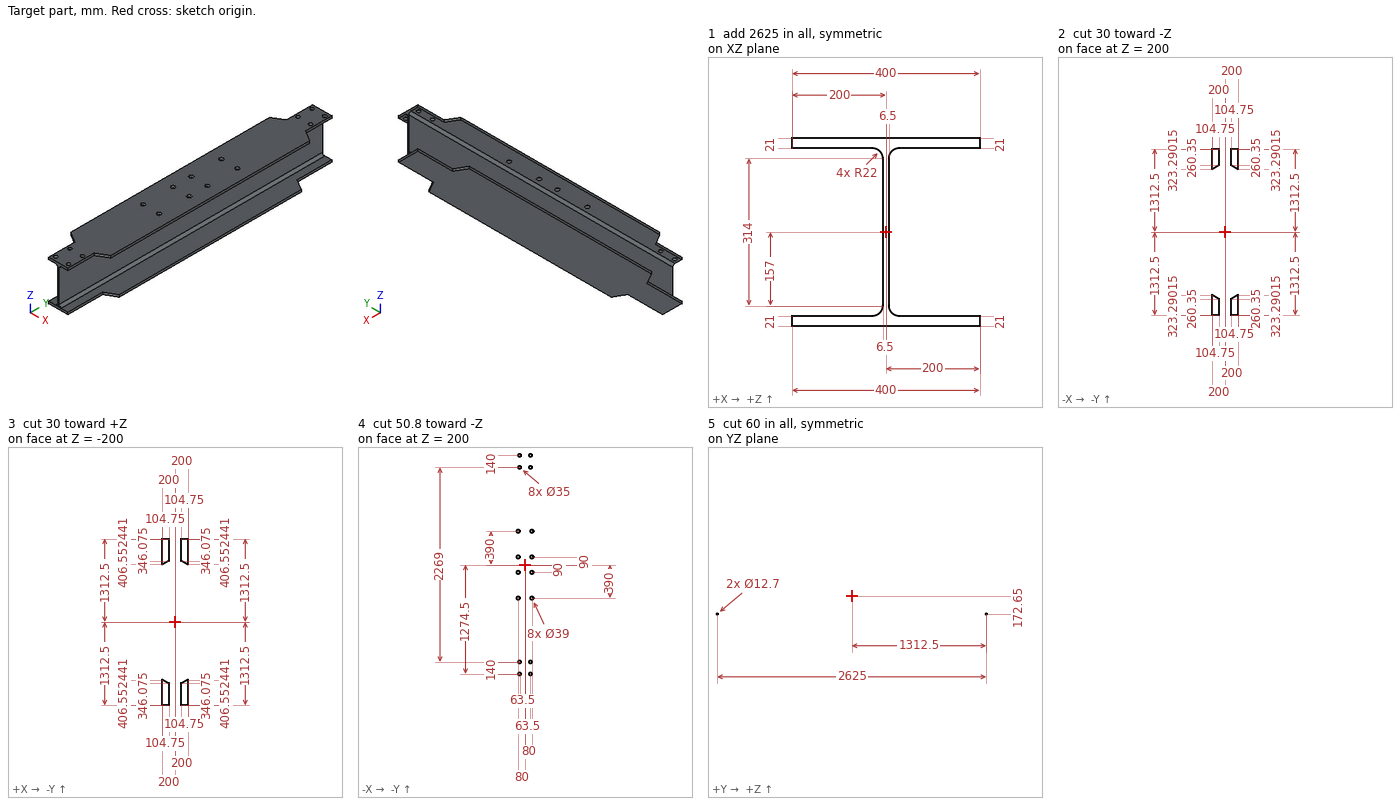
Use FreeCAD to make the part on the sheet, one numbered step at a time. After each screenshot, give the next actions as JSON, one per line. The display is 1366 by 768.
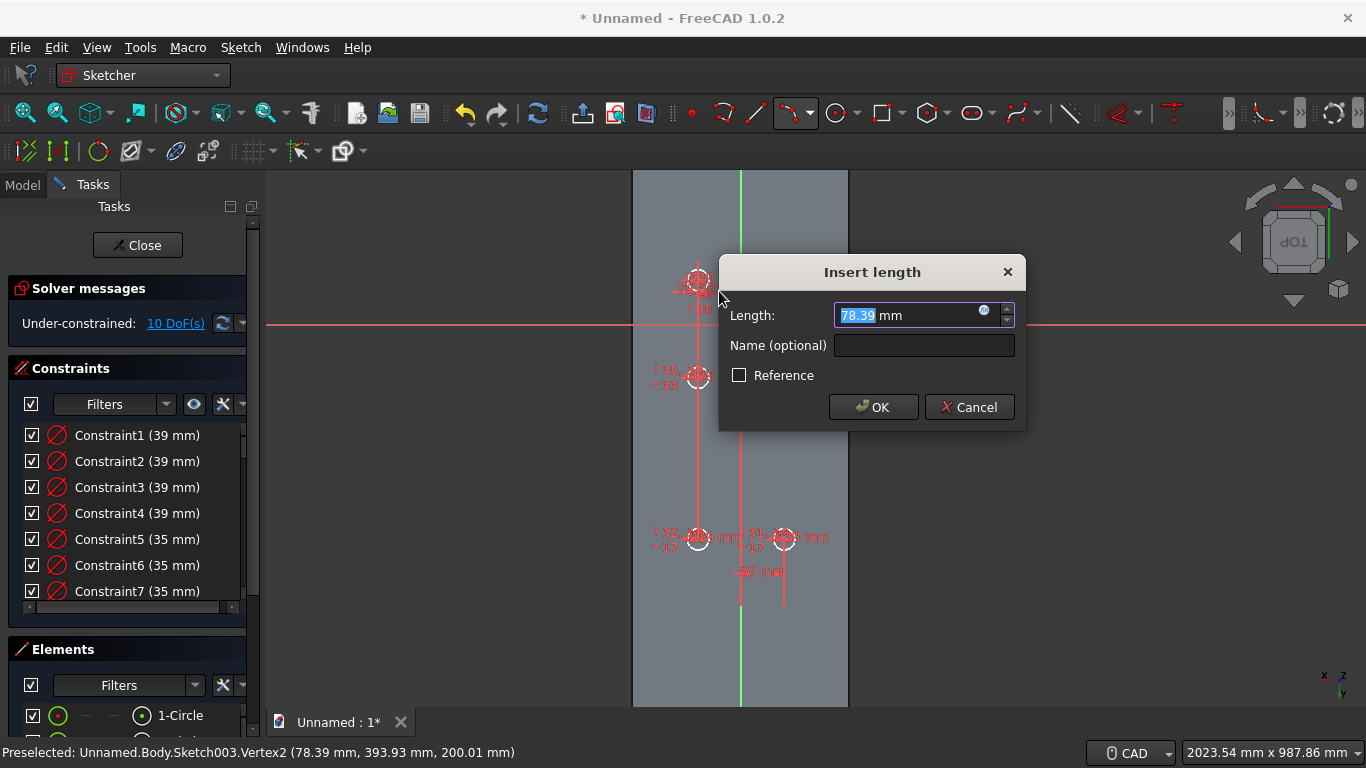
{"action": "type", "text": "80"}
{"action": "key", "text": "Return"}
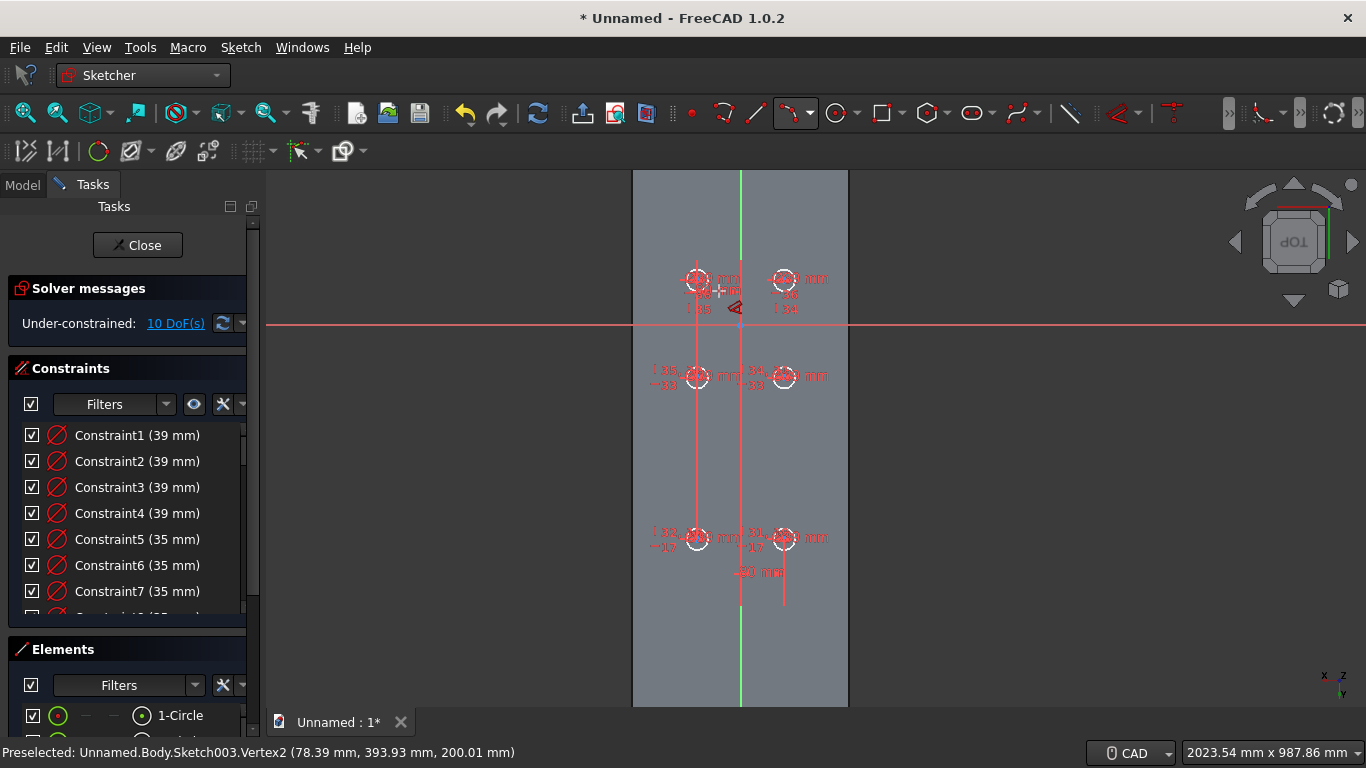
{"action": "left_click", "coordinate": [784, 378]}
{"action": "left_click", "coordinate": [818, 352]}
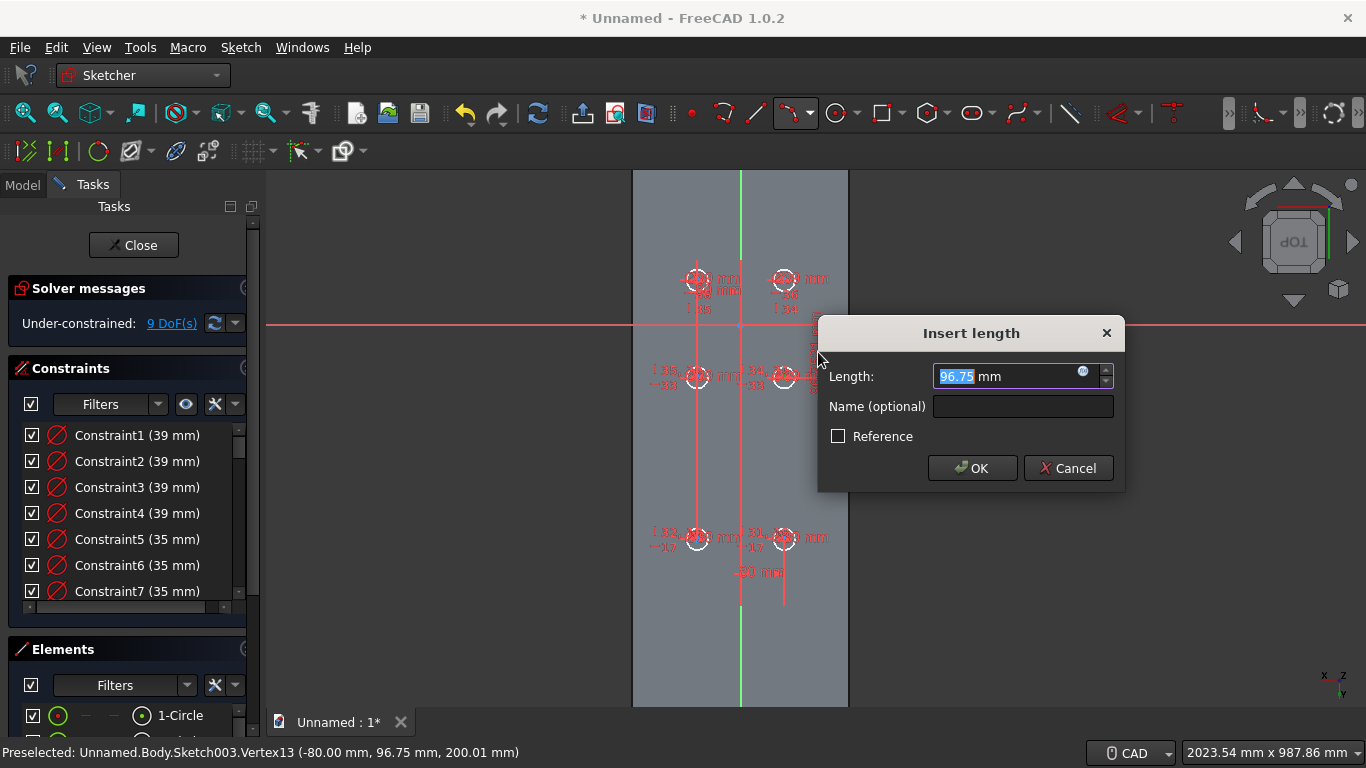
{"action": "type", "text": "90"}
{"action": "key", "text": "Return"}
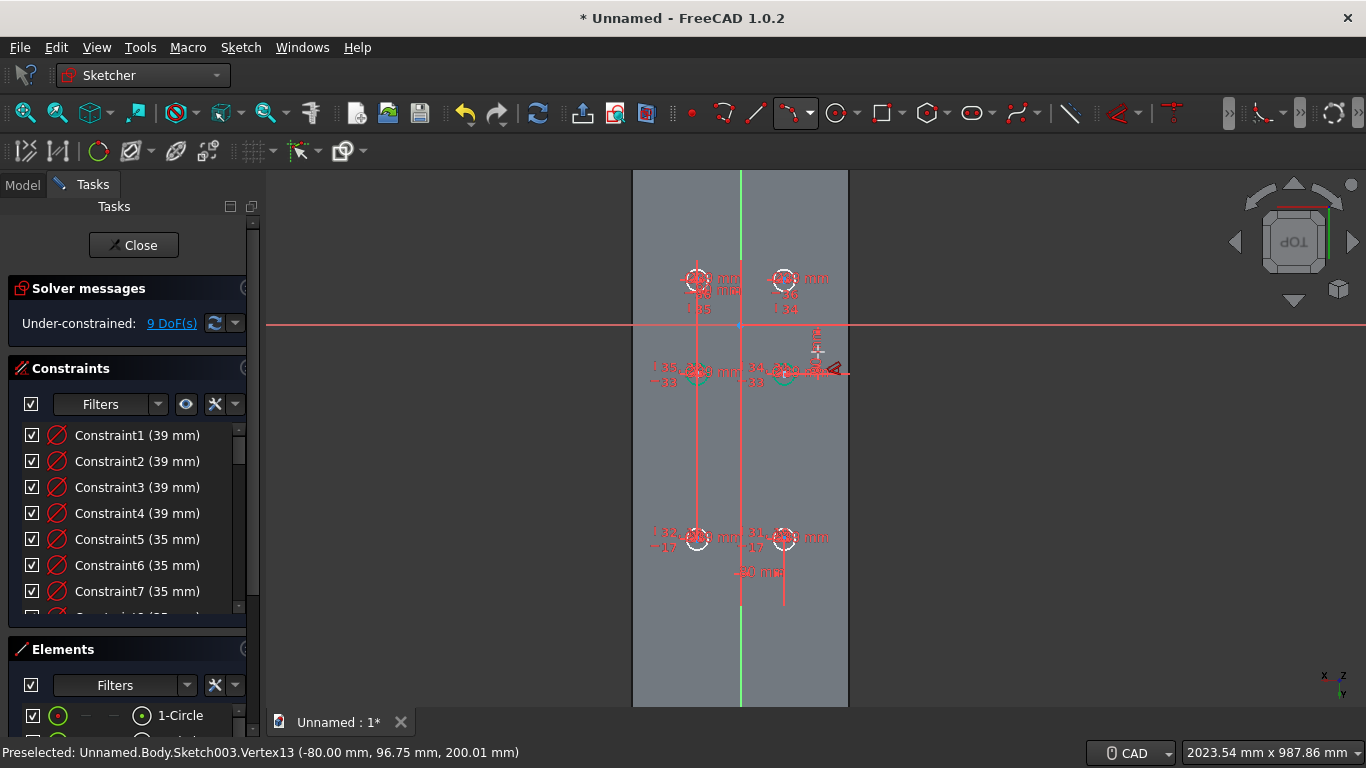
{"action": "left_click", "coordinate": [784, 280]}
{"action": "left_click", "coordinate": [818, 303]}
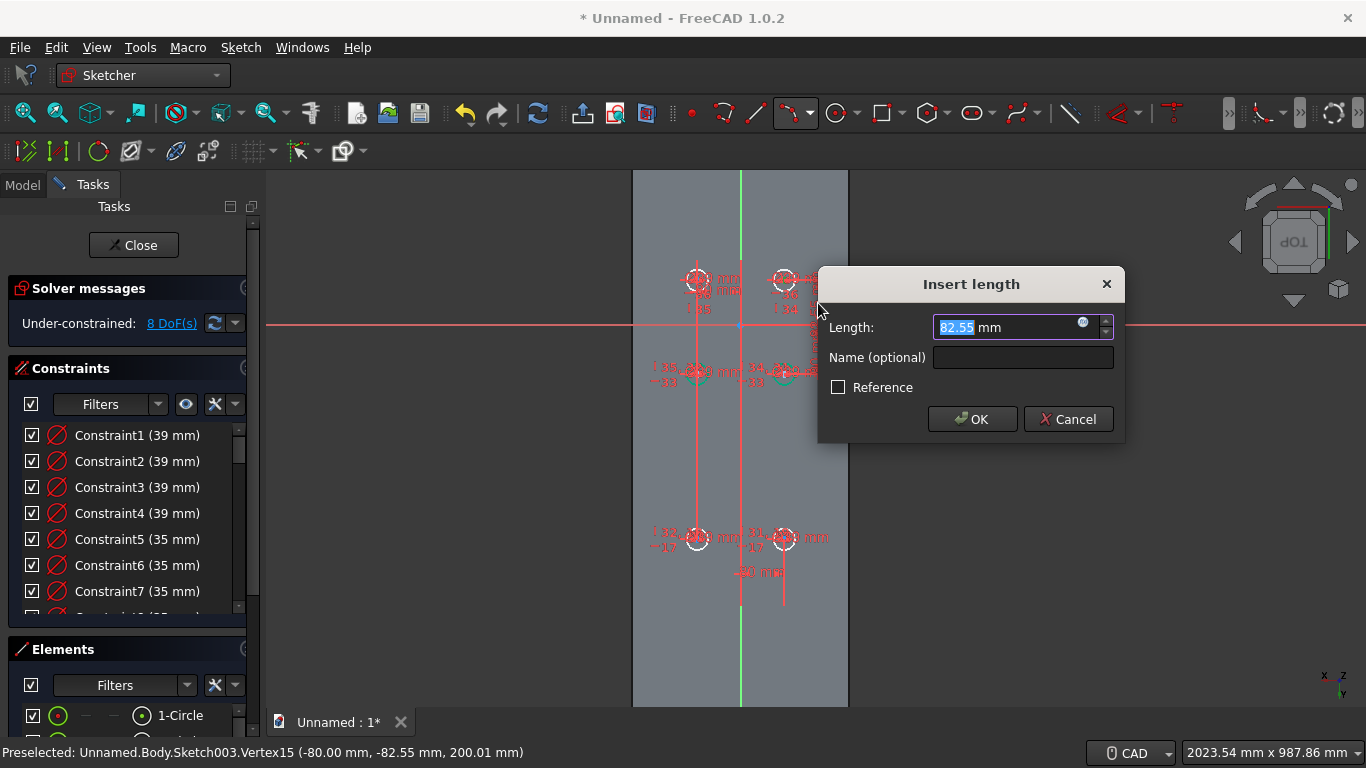
{"action": "type", "text": "90"}
{"action": "key", "text": "Return"}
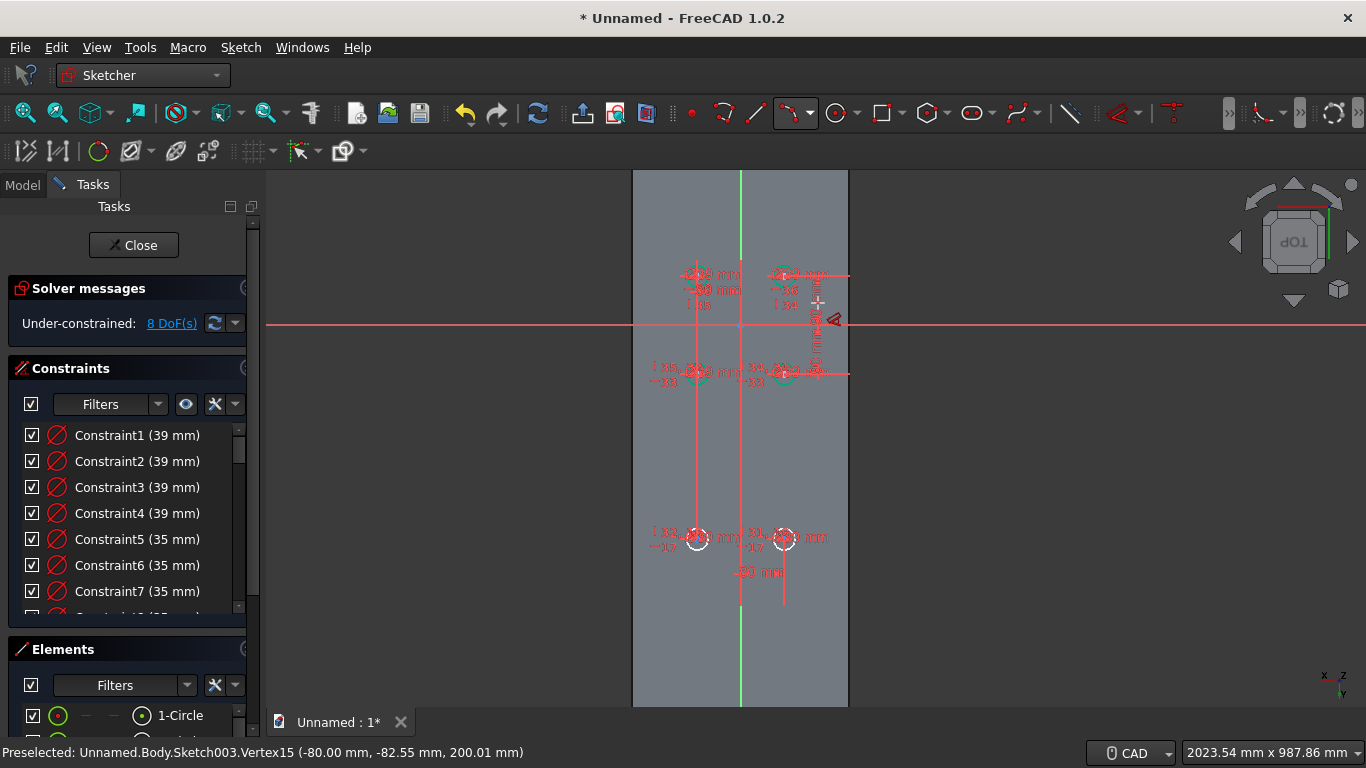
{"action": "scroll", "coordinate": [750, 476], "scroll_direction": "down", "scroll_amount": 7}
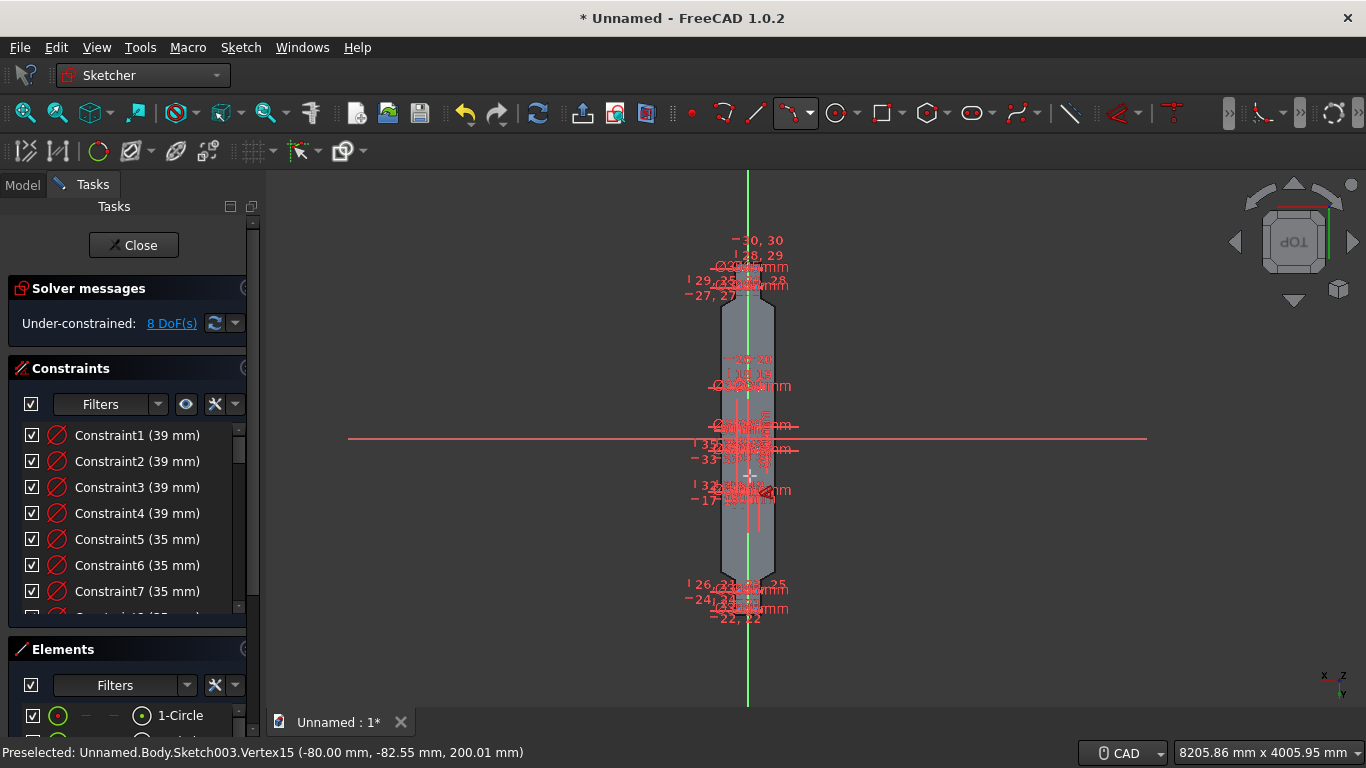
{"action": "left_click", "coordinate": [759, 492]}
{"action": "left_click", "coordinate": [793, 478]}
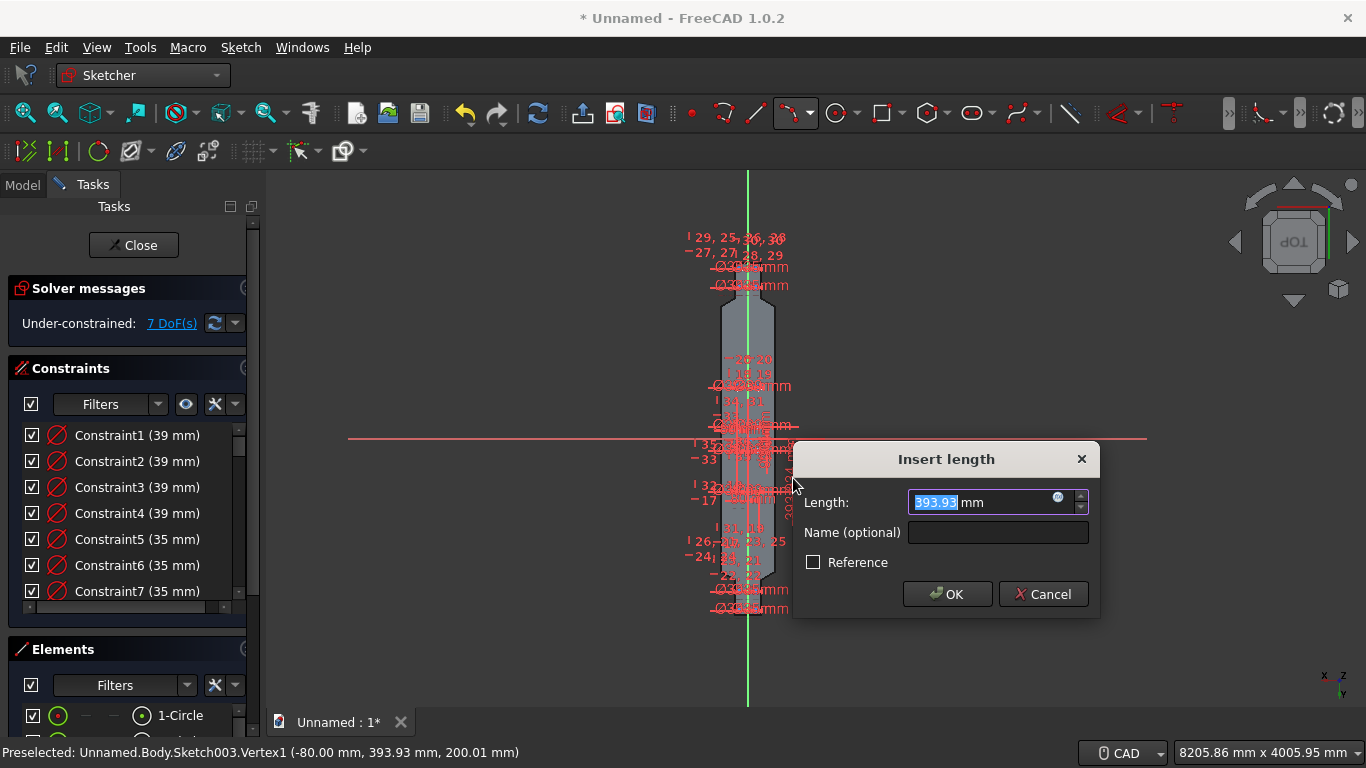
{"action": "type", "text": "390"}
{"action": "key", "text": "Return"}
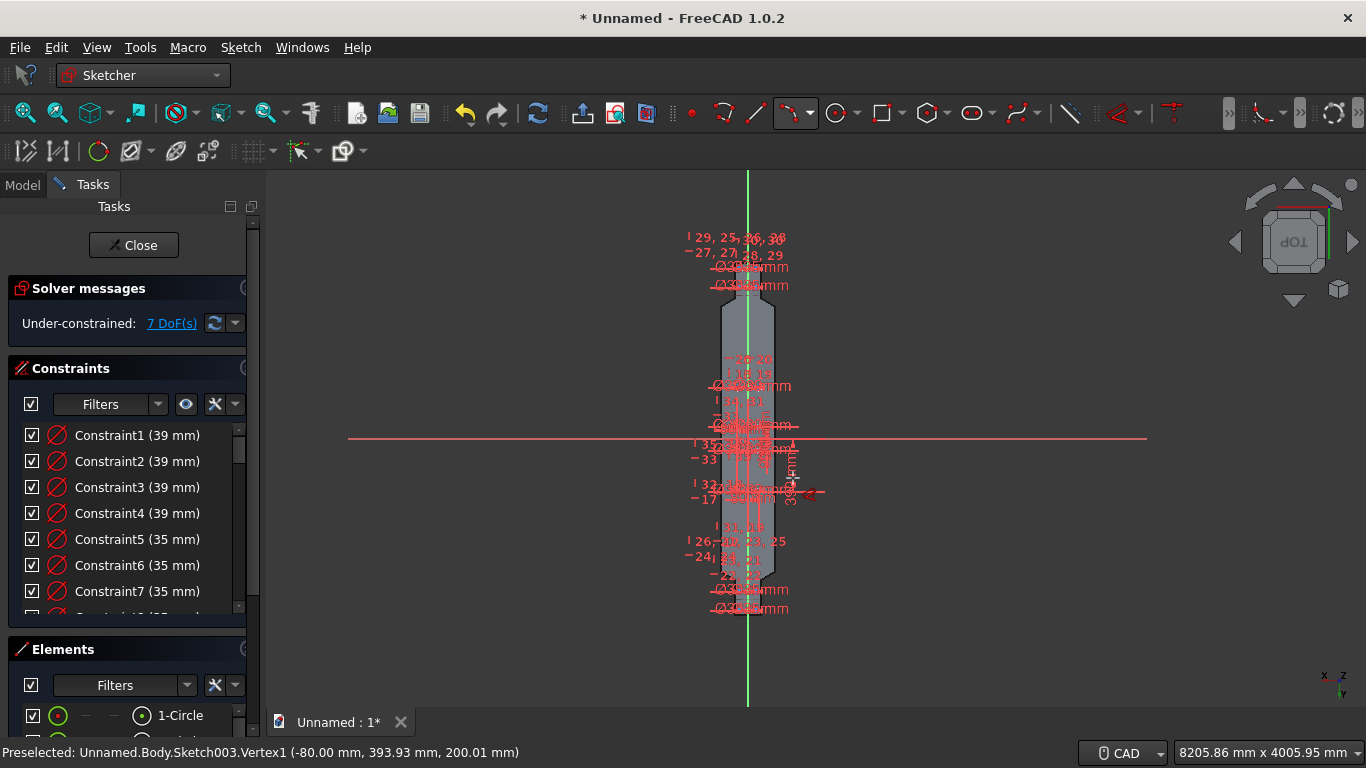
{"action": "left_click", "coordinate": [737, 388]}
{"action": "left_click", "coordinate": [703, 402]}